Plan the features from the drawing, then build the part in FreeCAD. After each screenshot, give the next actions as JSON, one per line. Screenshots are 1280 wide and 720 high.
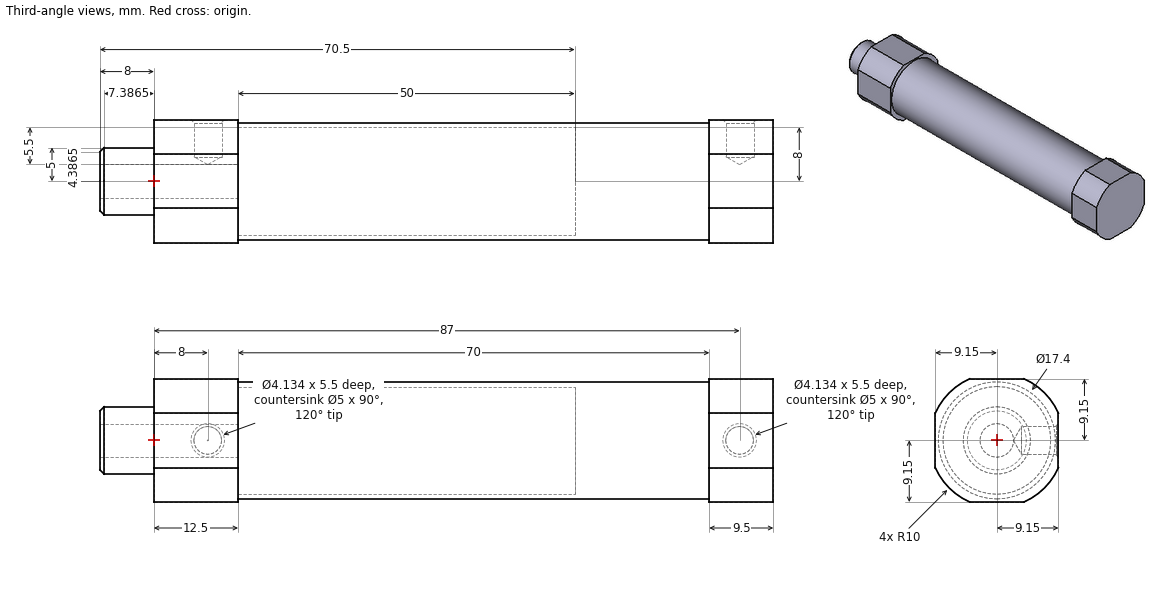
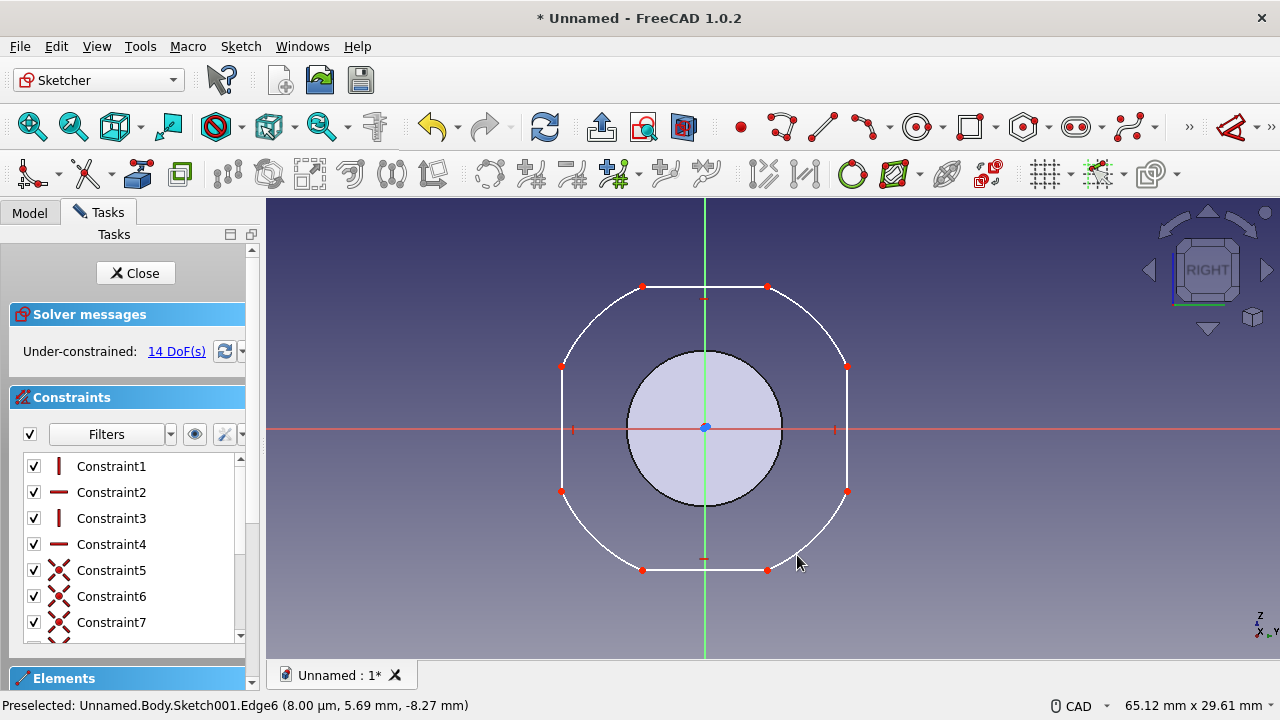
{"action": "left_click", "coordinate": [580, 521]}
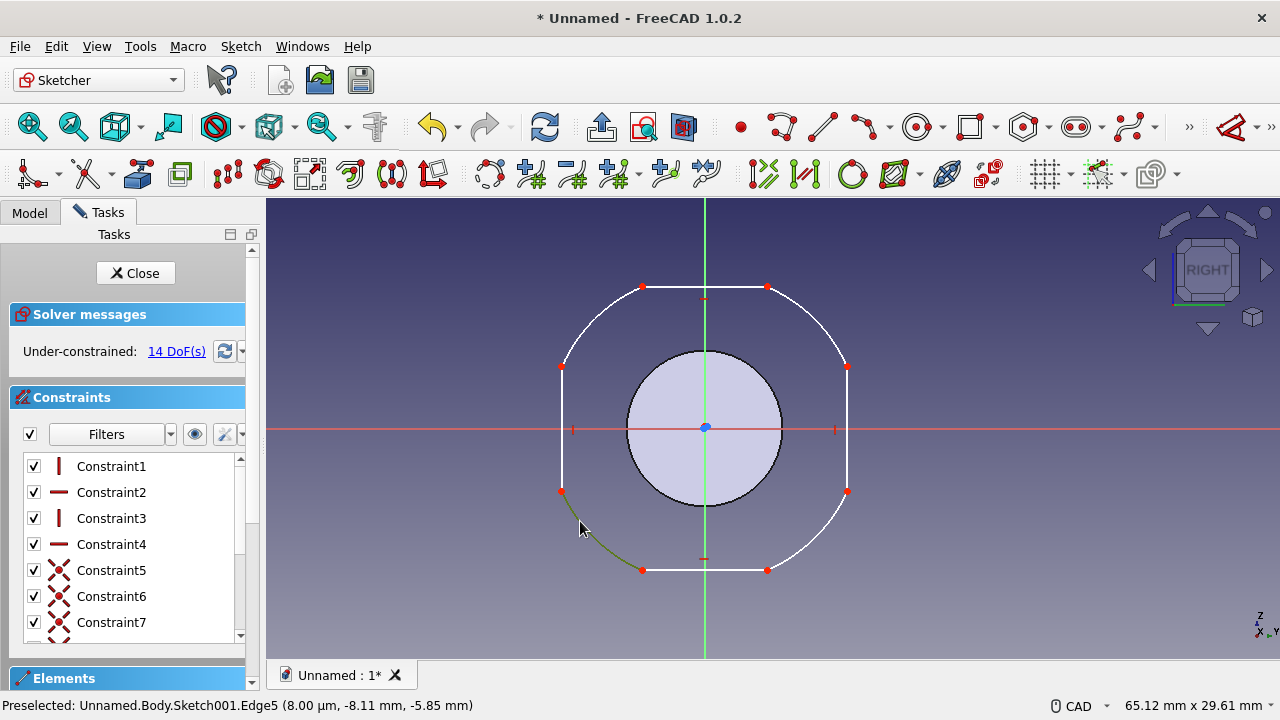
{"action": "left_click", "coordinate": [830, 337]}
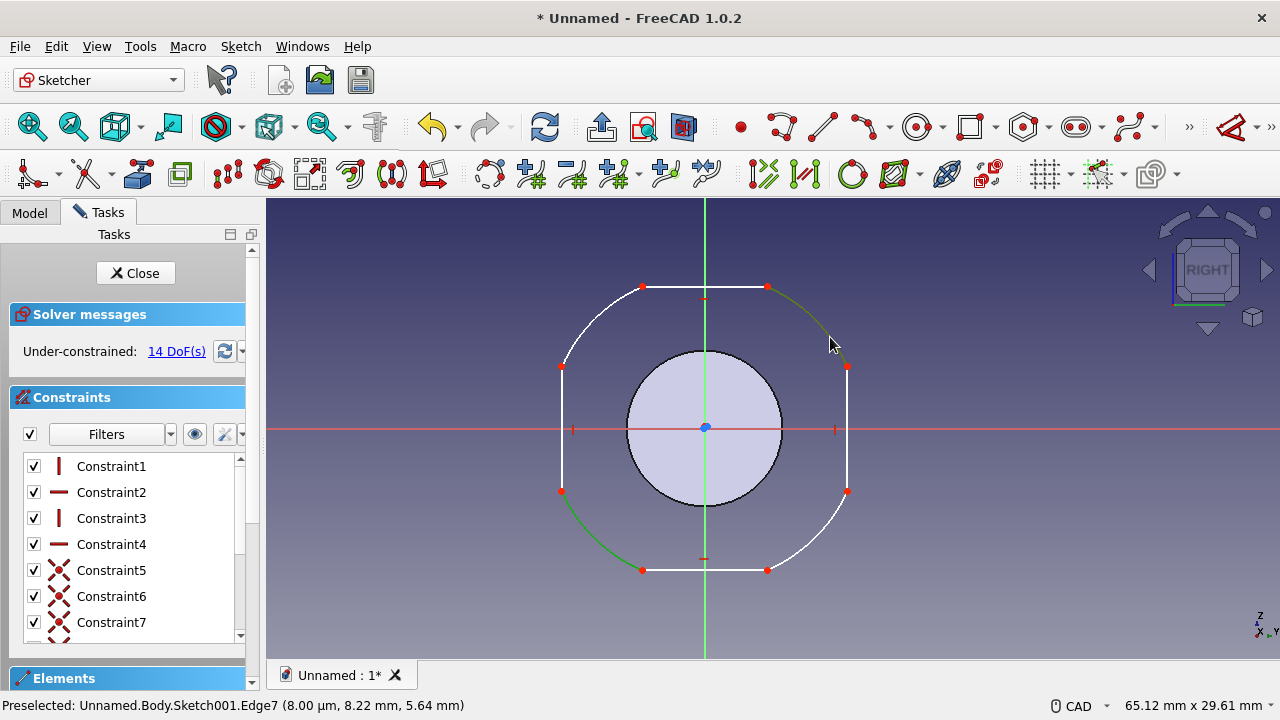
{"action": "key", "text": "c"}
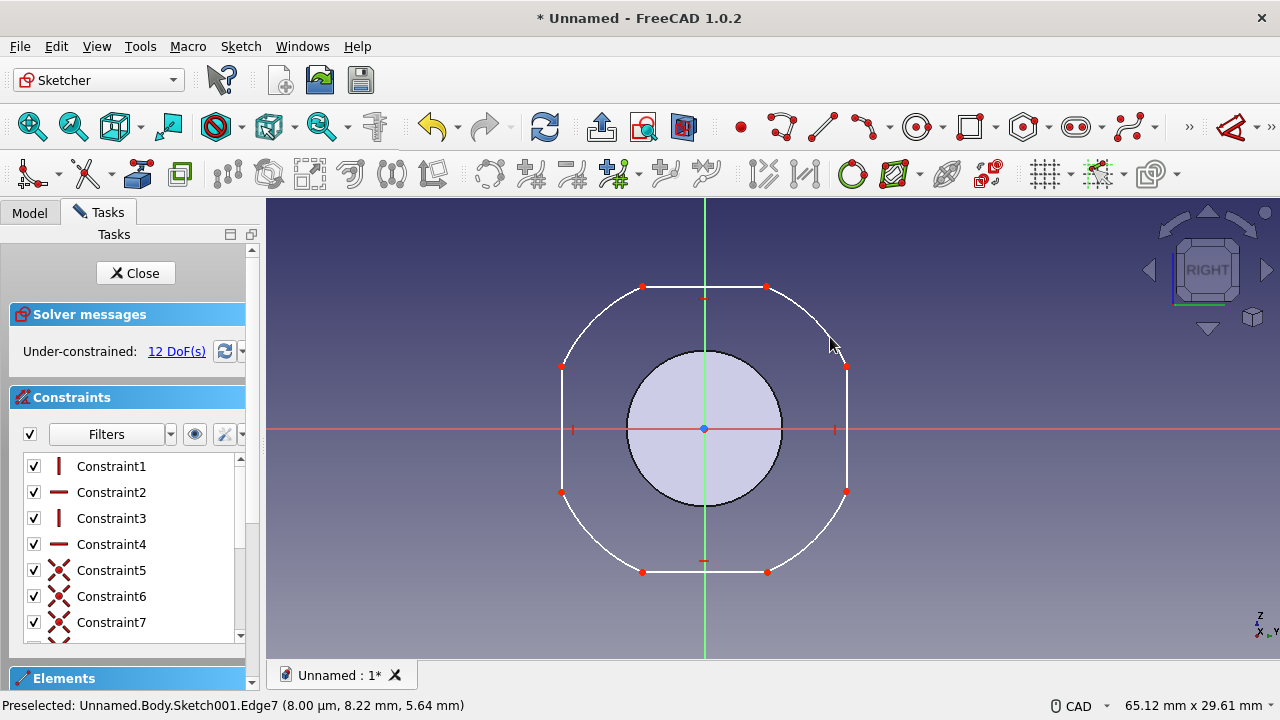
{"action": "left_click", "coordinate": [579, 522]}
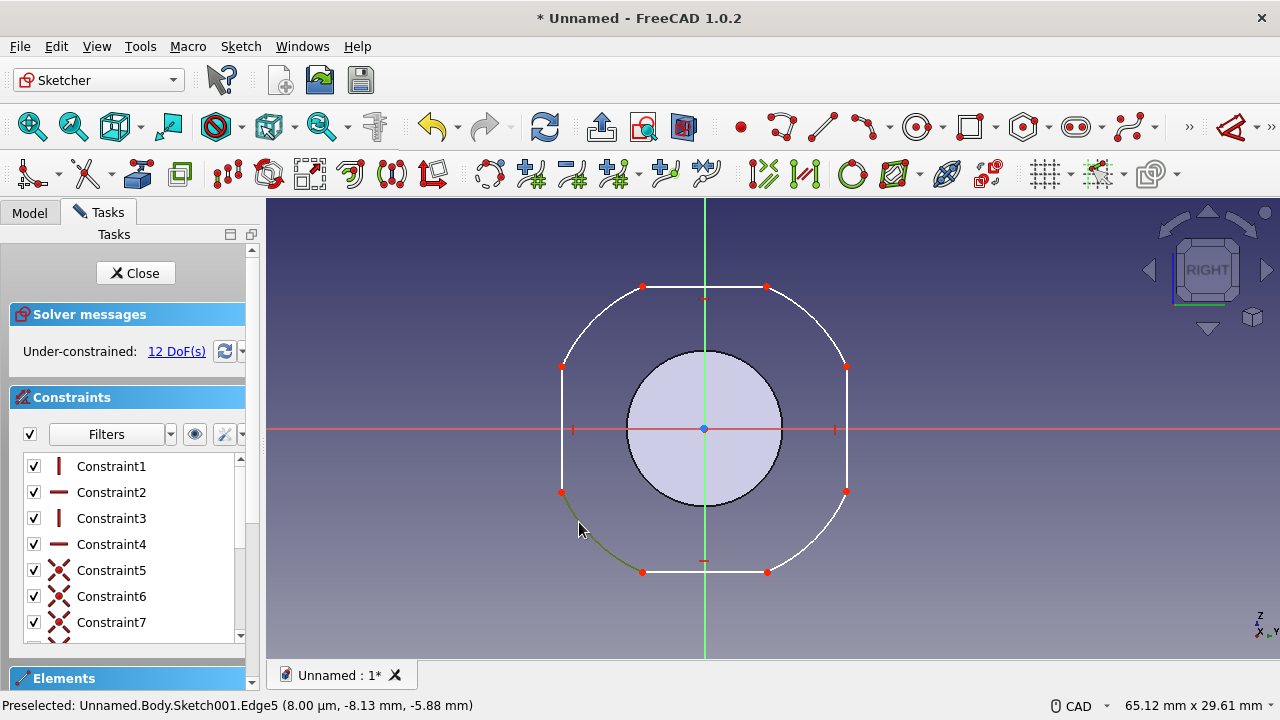
{"action": "left_click", "coordinate": [612, 304]}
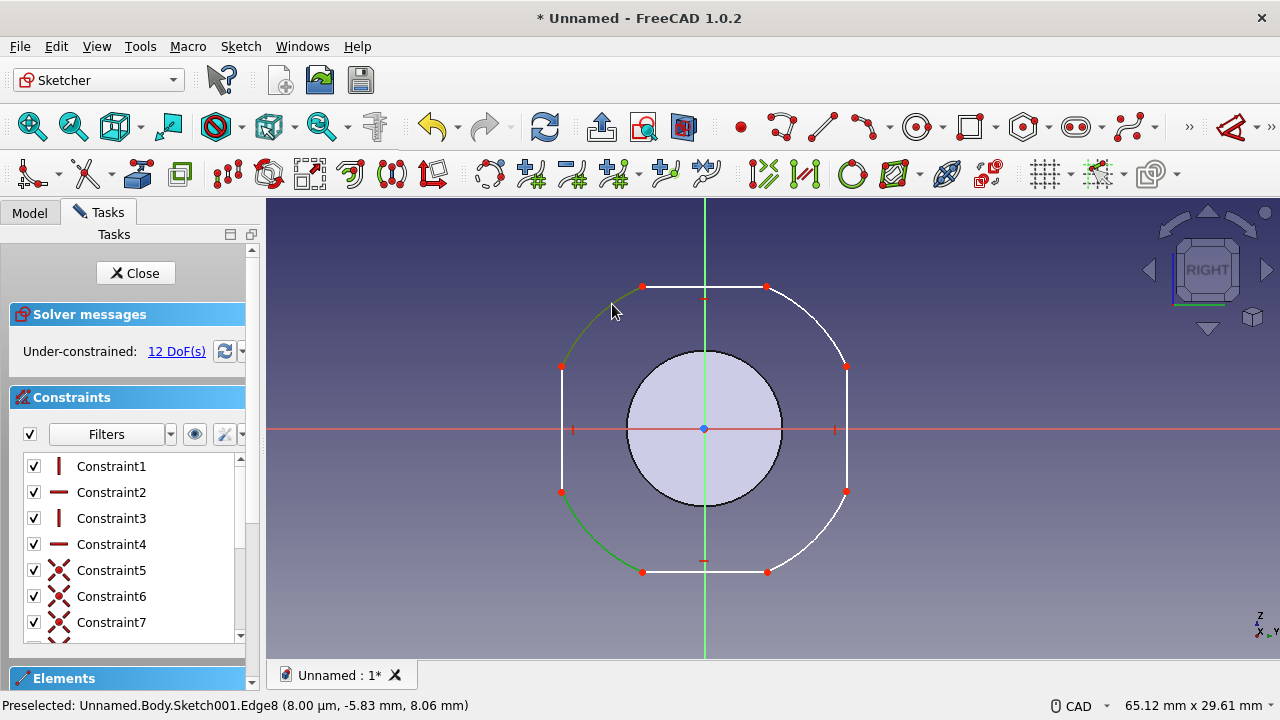
{"action": "key", "text": "c"}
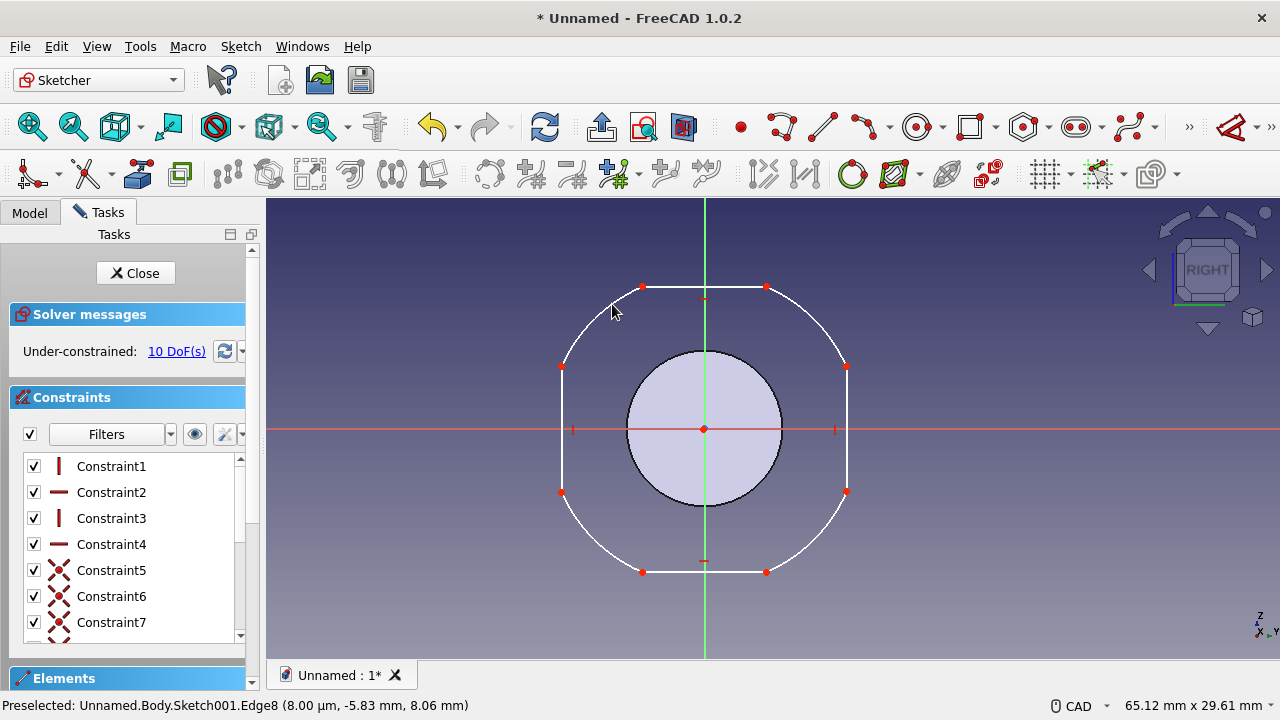
{"action": "left_click_drag", "start_coordinate": [694, 418], "coordinate": [715, 439]}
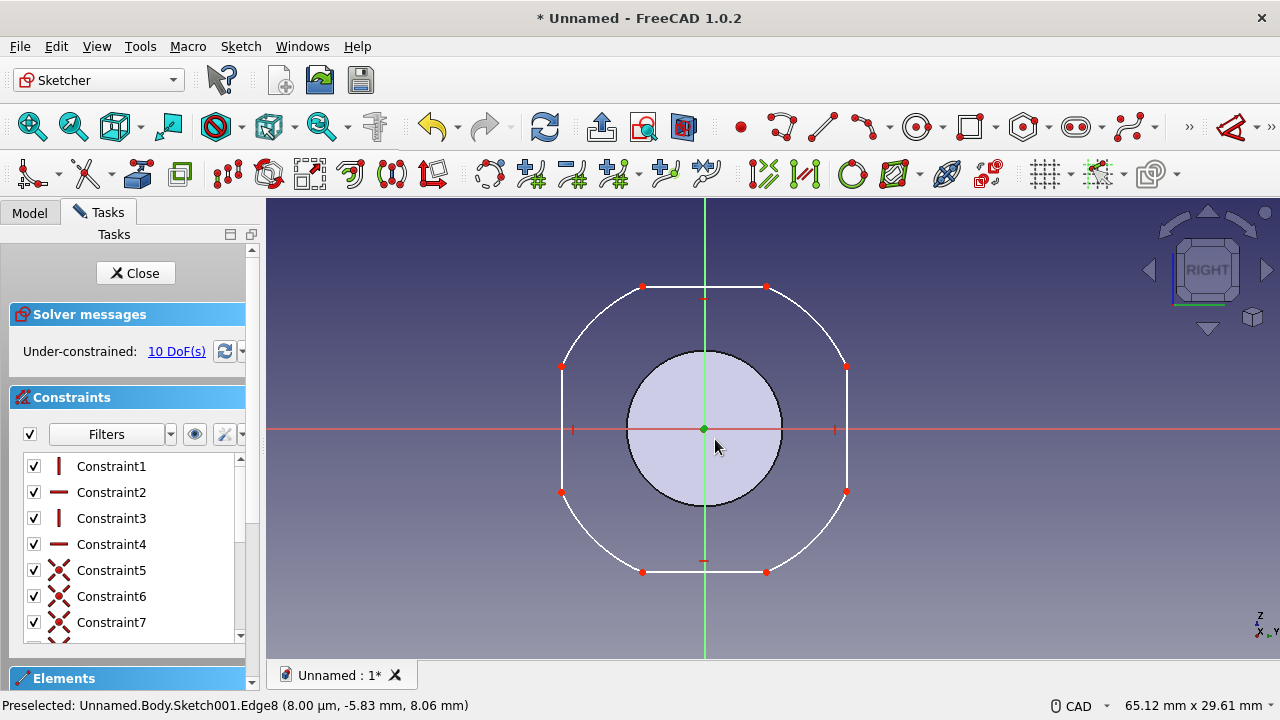
{"action": "key", "text": "c"}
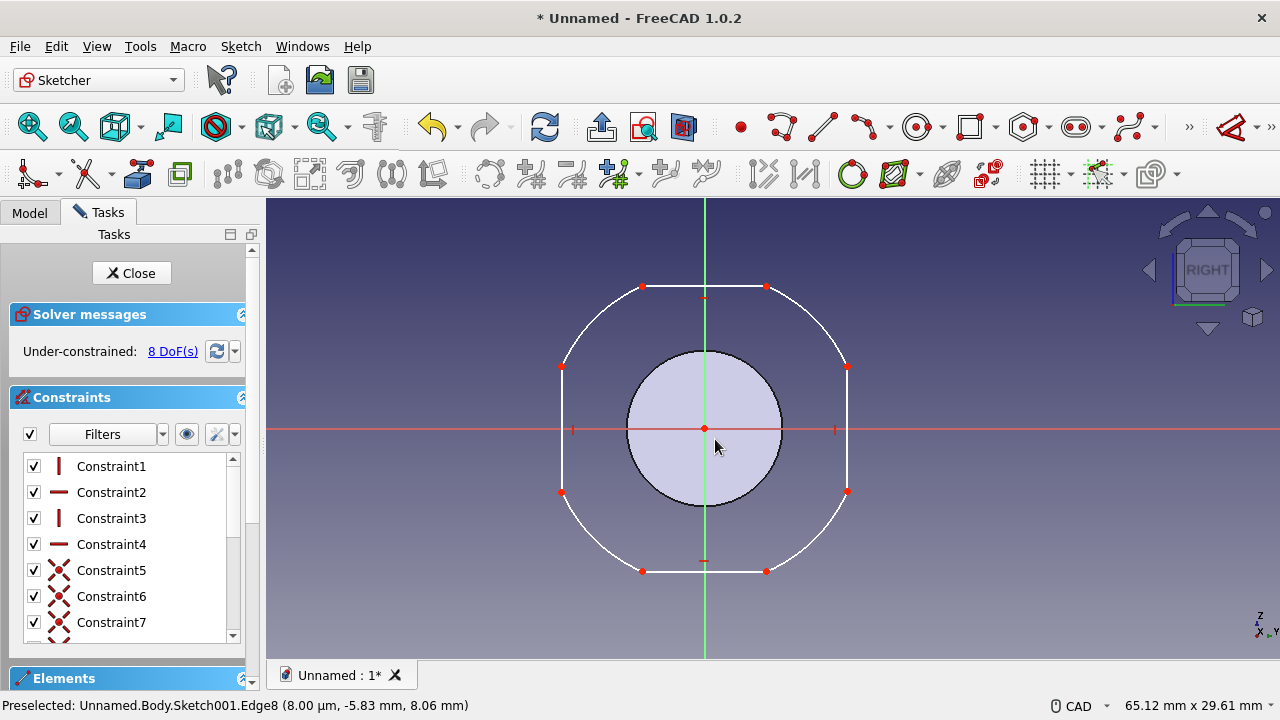
{"action": "left_click", "coordinate": [579, 522]}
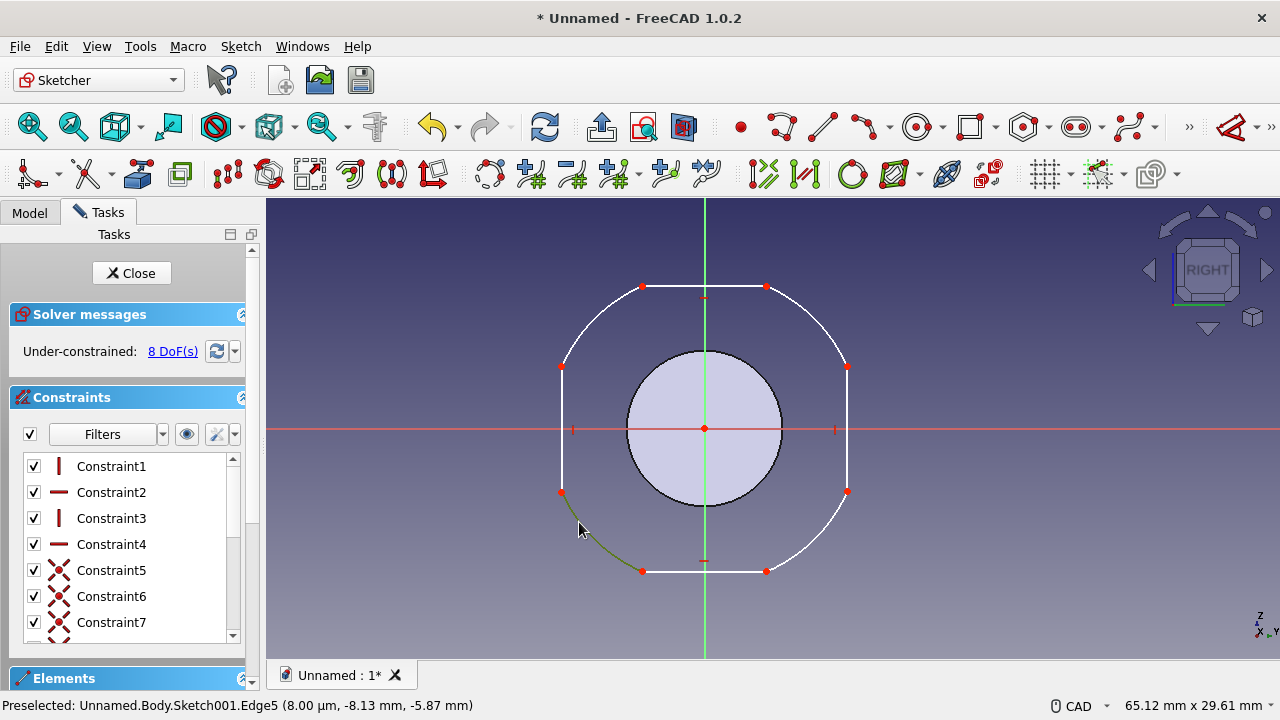
{"action": "left_click", "coordinate": [797, 554]}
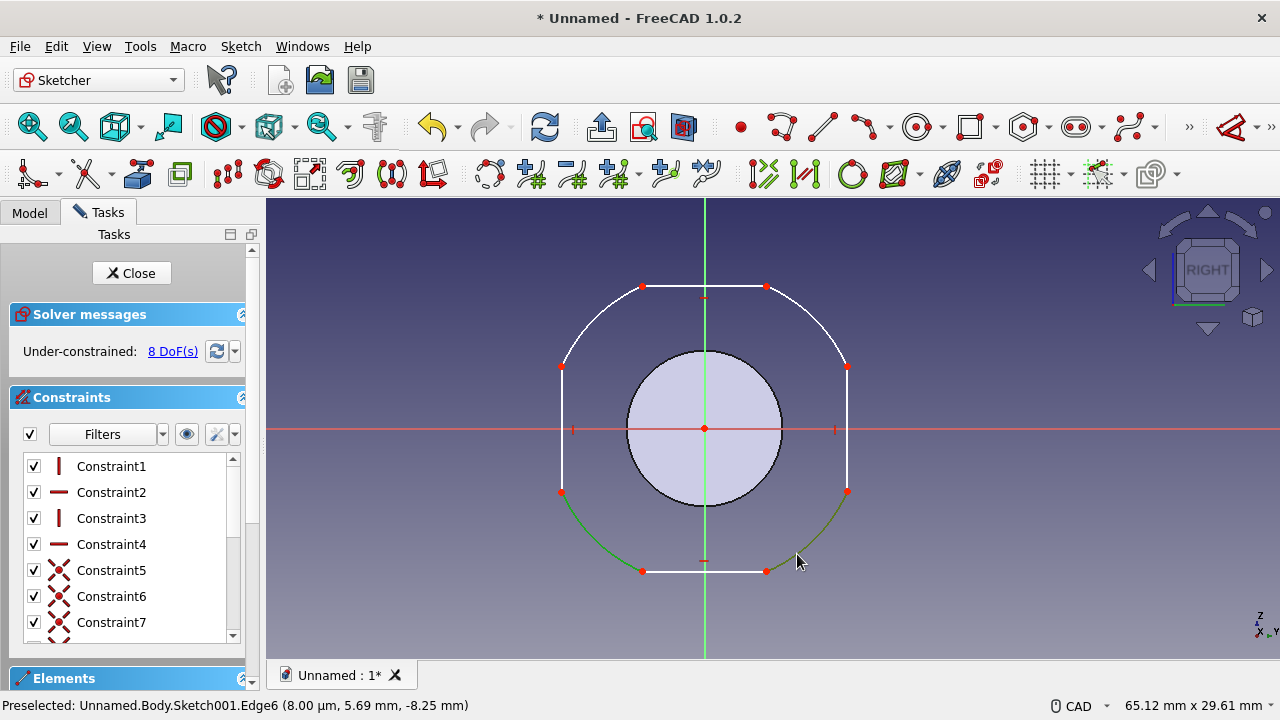
{"action": "left_click", "coordinate": [830, 337]}